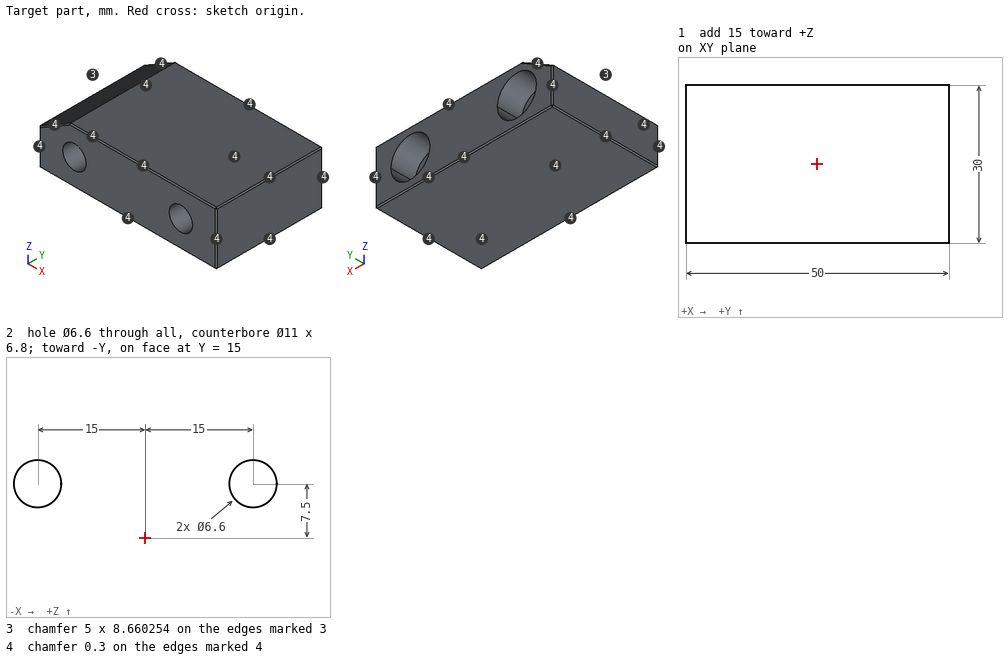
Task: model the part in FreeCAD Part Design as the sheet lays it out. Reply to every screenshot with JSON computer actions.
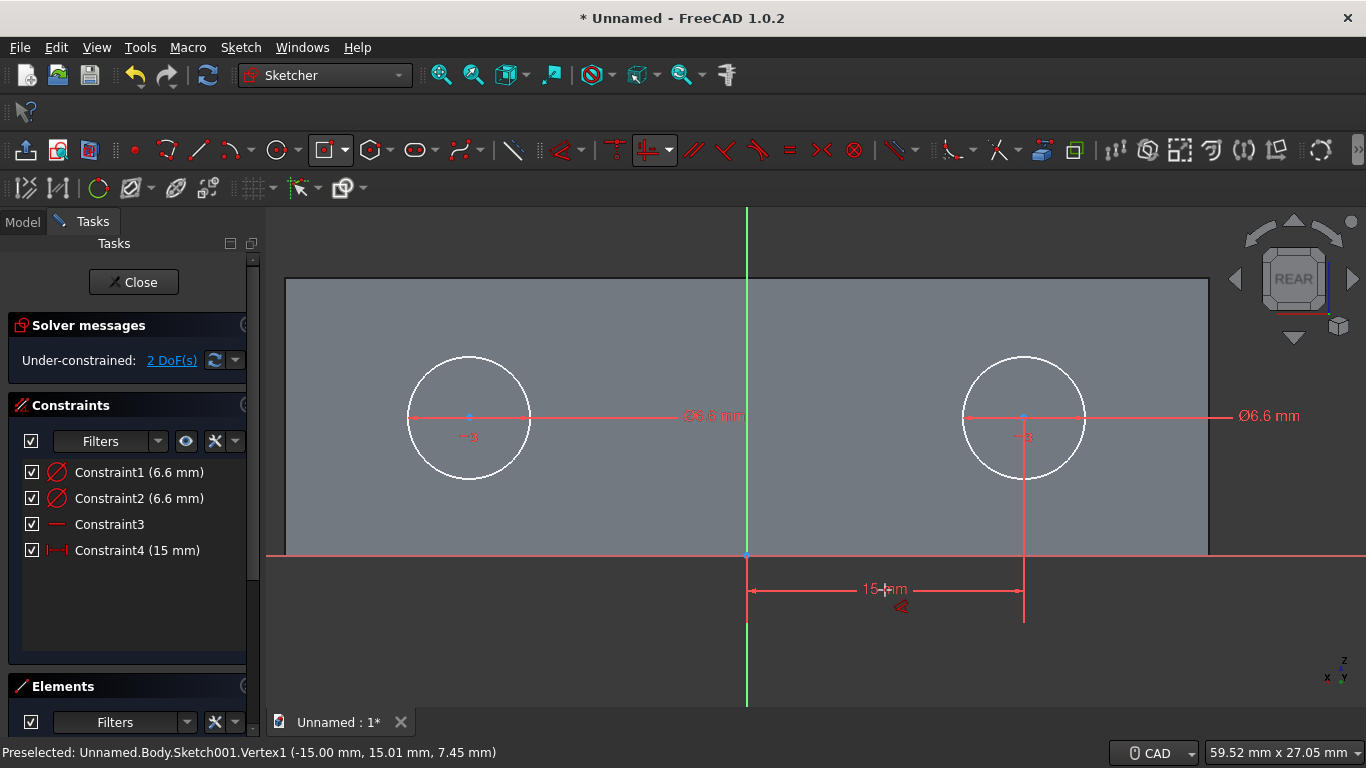
{"action": "left_click", "coordinate": [469, 418]}
{"action": "left_click", "coordinate": [608, 590]}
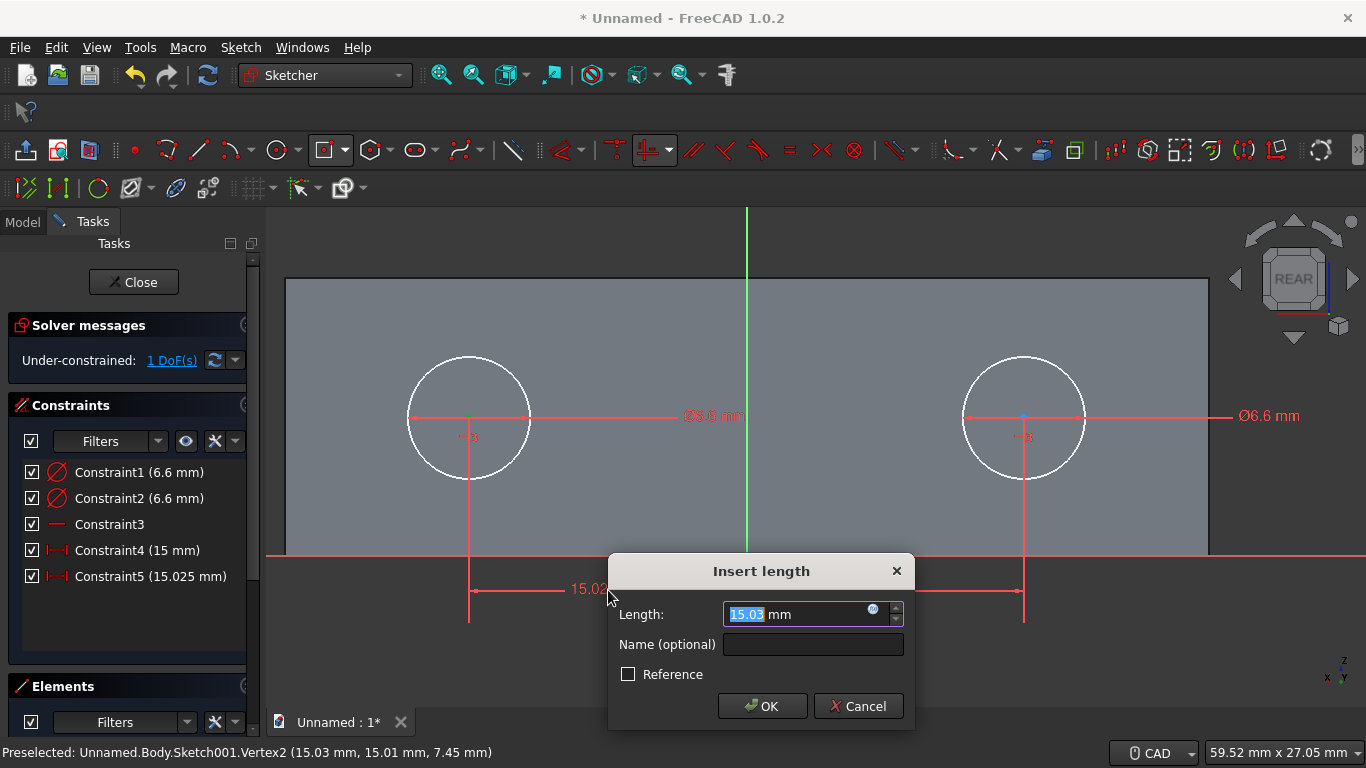
{"action": "type", "text": "15"}
{"action": "key", "text": "Return"}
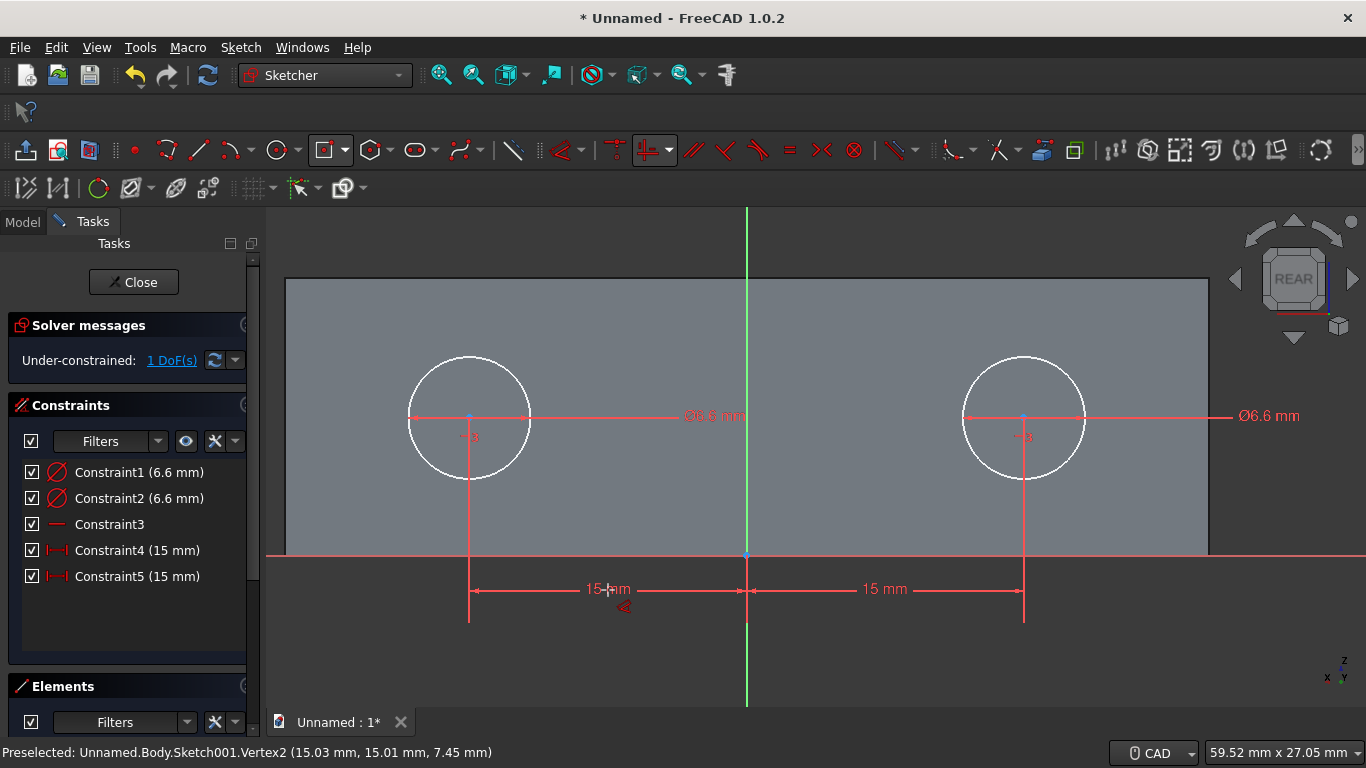
{"action": "left_click", "coordinate": [1024, 418]}
{"action": "left_click", "coordinate": [1058, 487]}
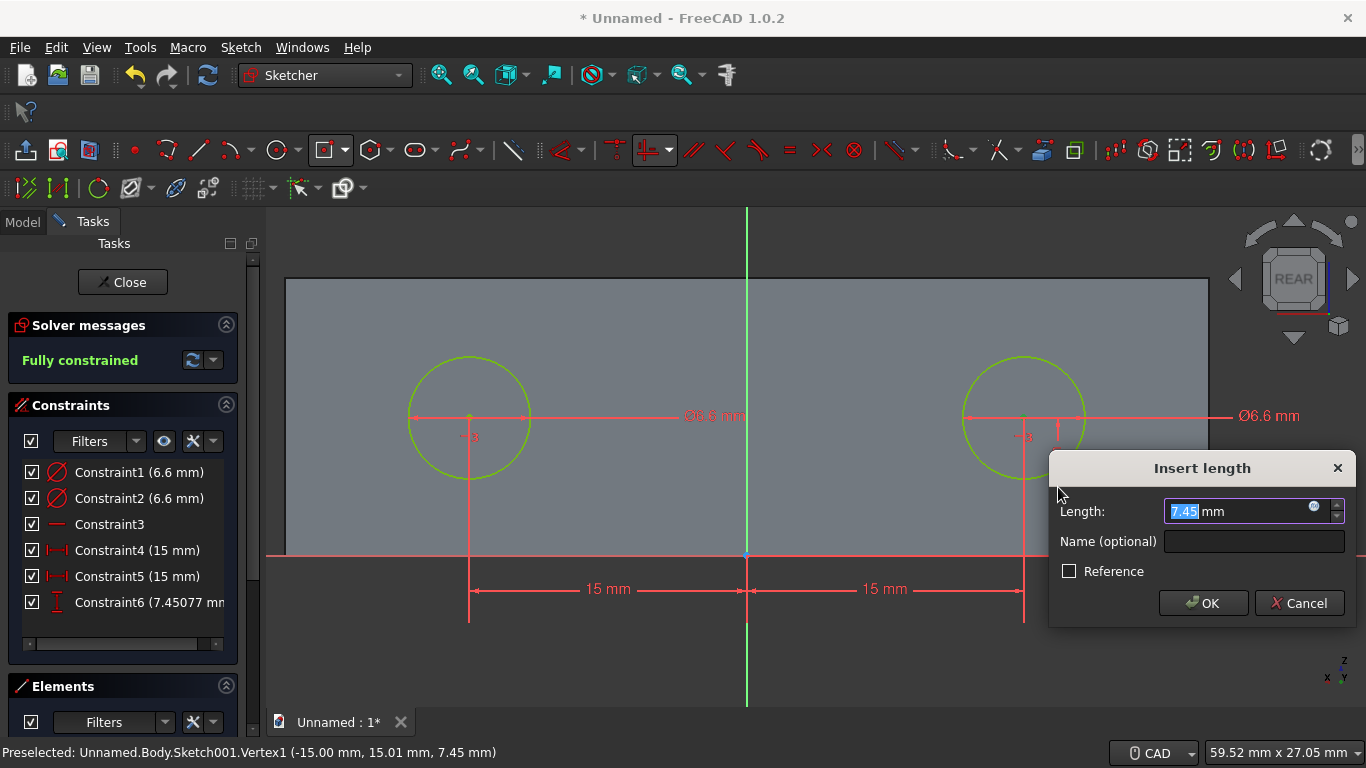
{"action": "type", "text": "7.5"}
{"action": "key", "text": "Return"}
{"action": "key", "text": "Escape"}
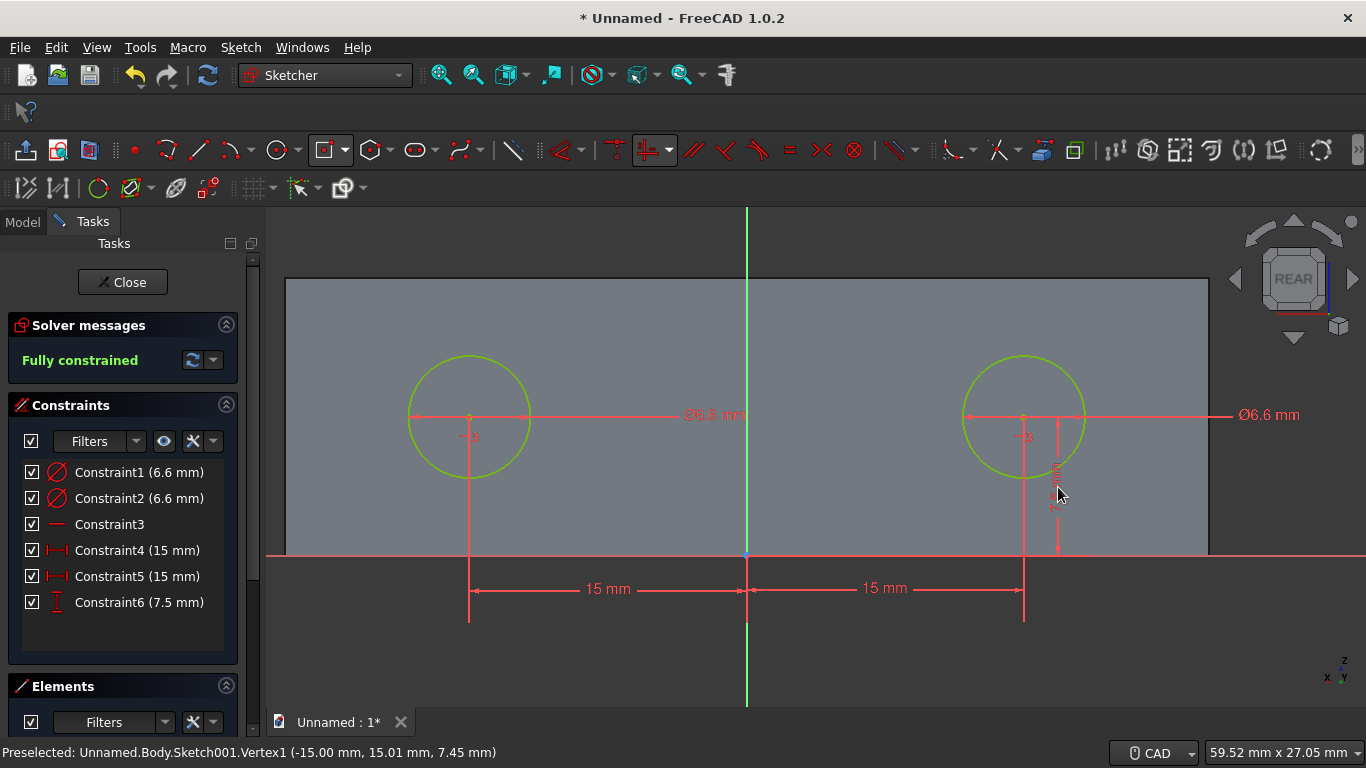
{"action": "left_click", "coordinate": [123, 282]}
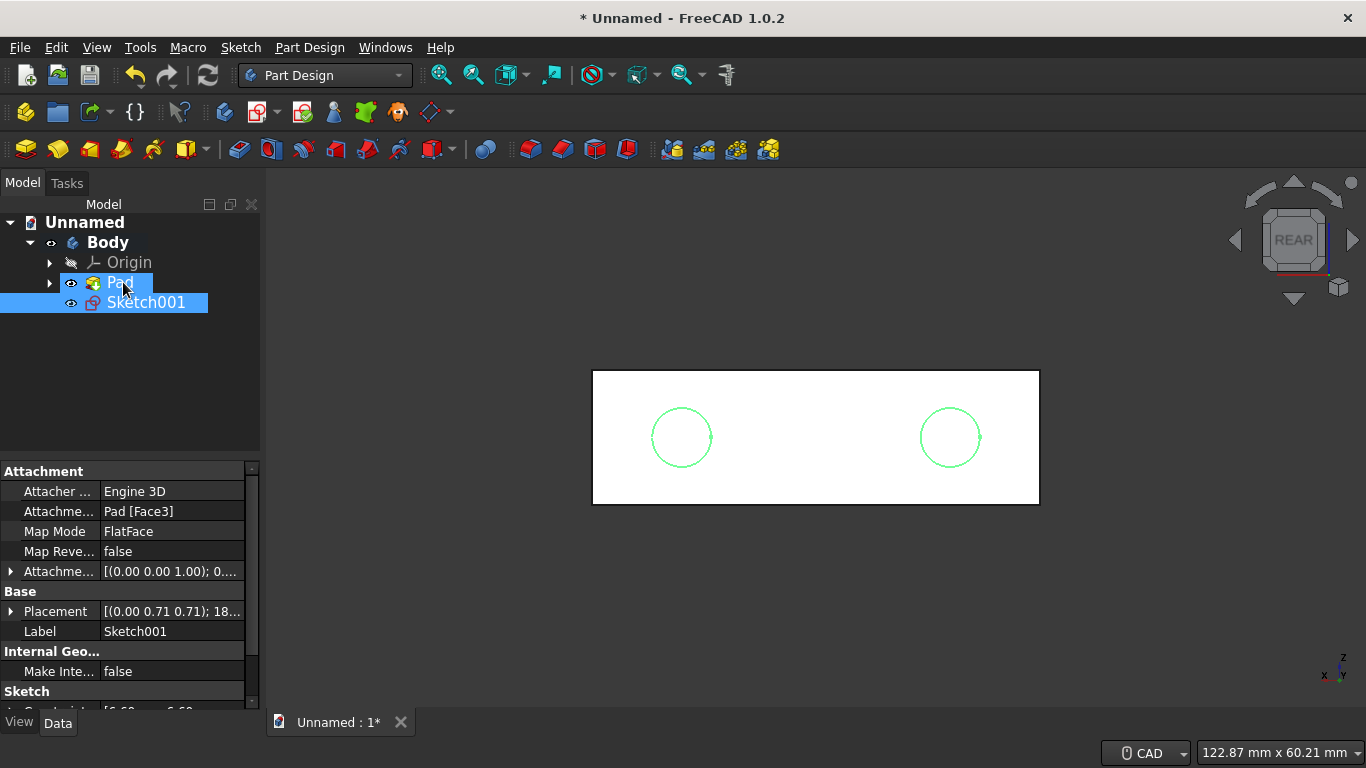
{"action": "left_click", "coordinate": [272, 150]}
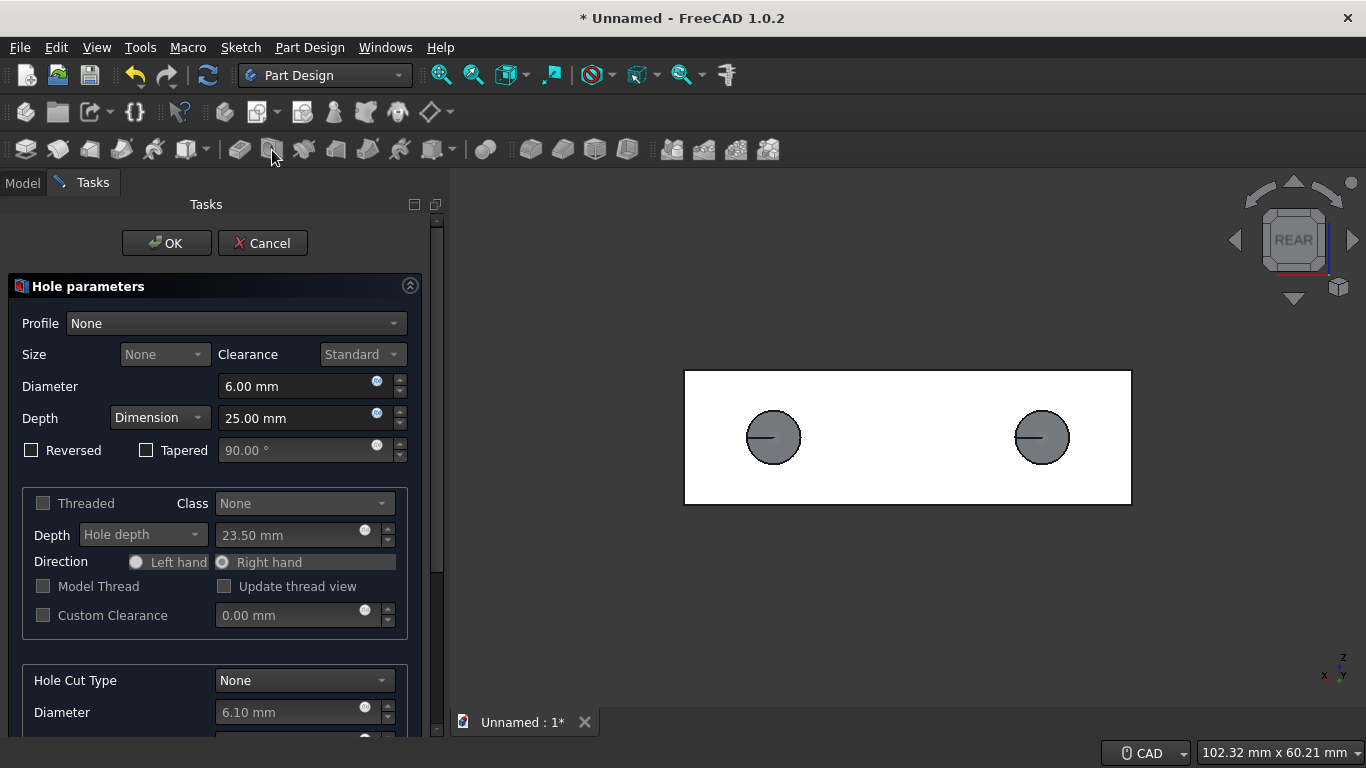
{"action": "triple_click", "coordinate": [305, 386]}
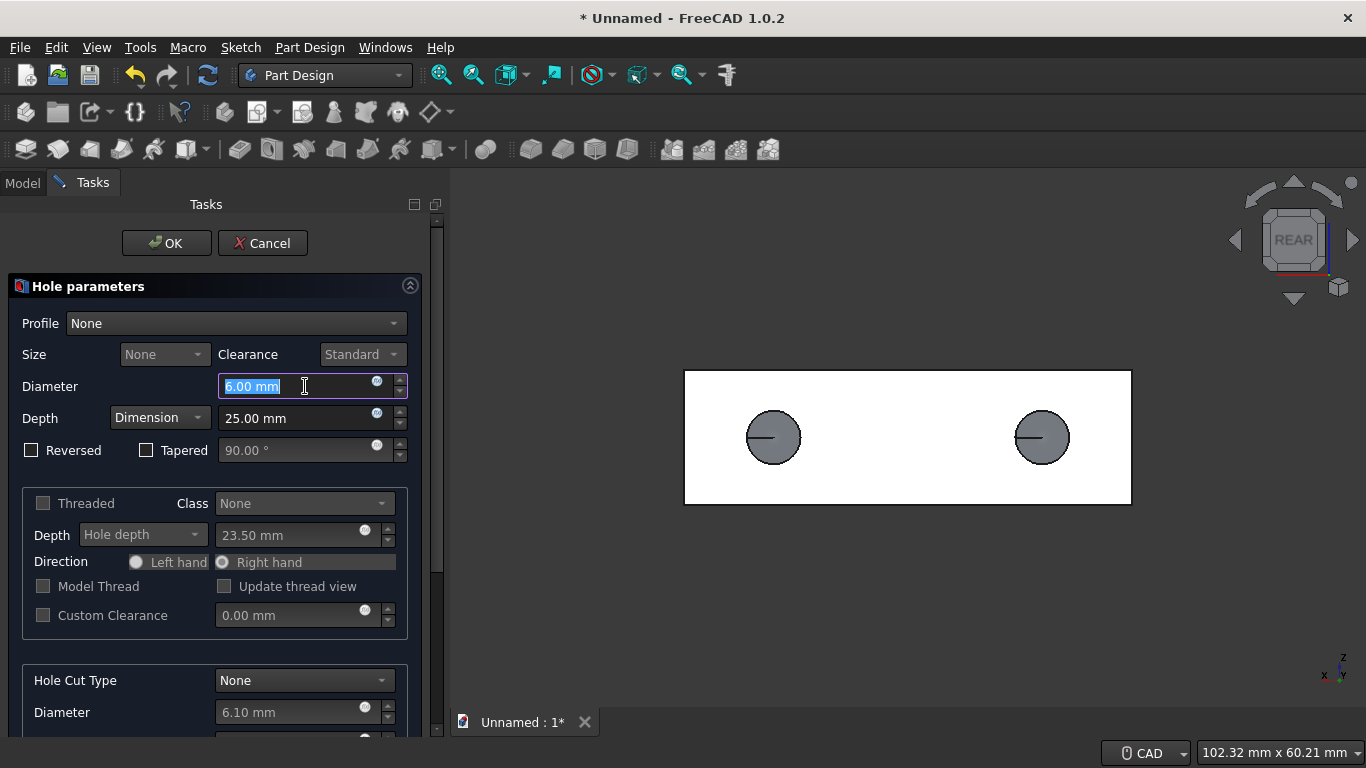
{"action": "type", "text": "6.6"}
{"action": "key", "text": "Tab"}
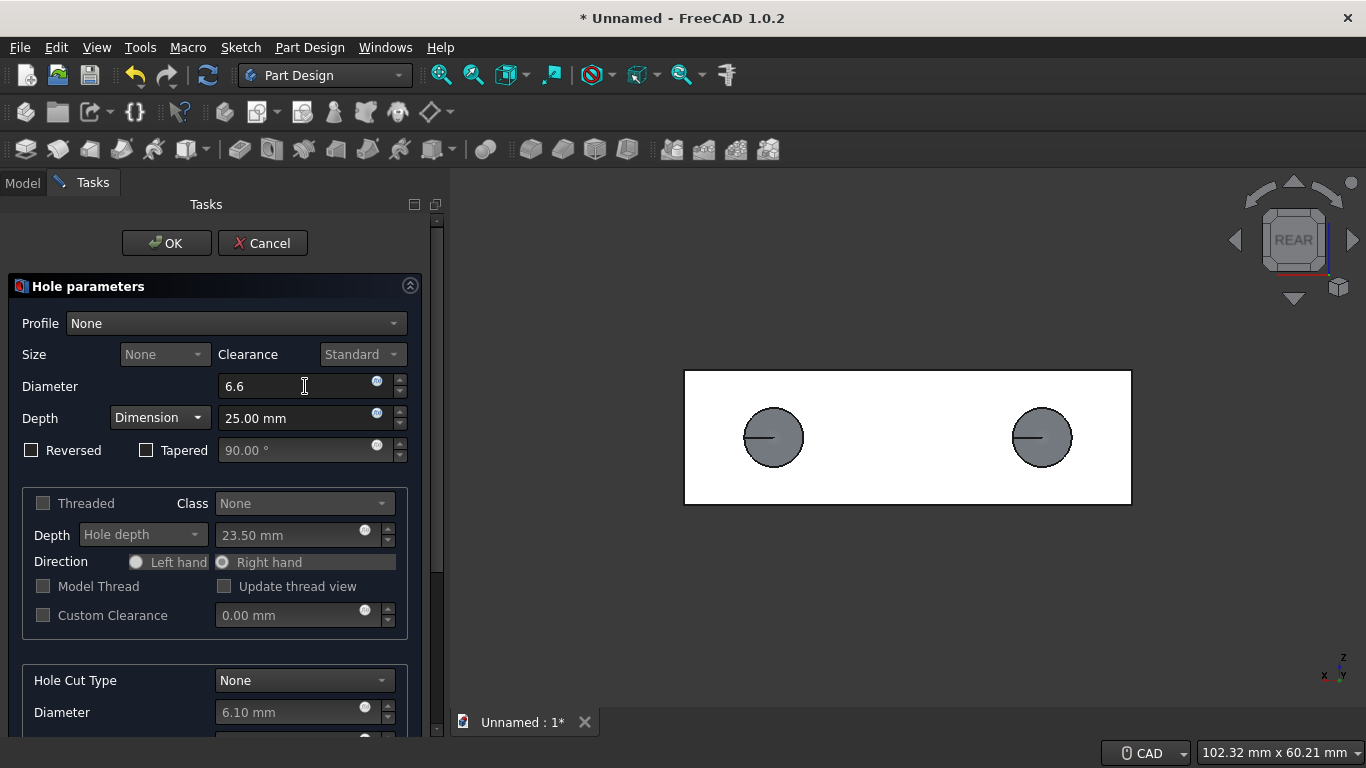
{"action": "left_click", "coordinate": [161, 418]}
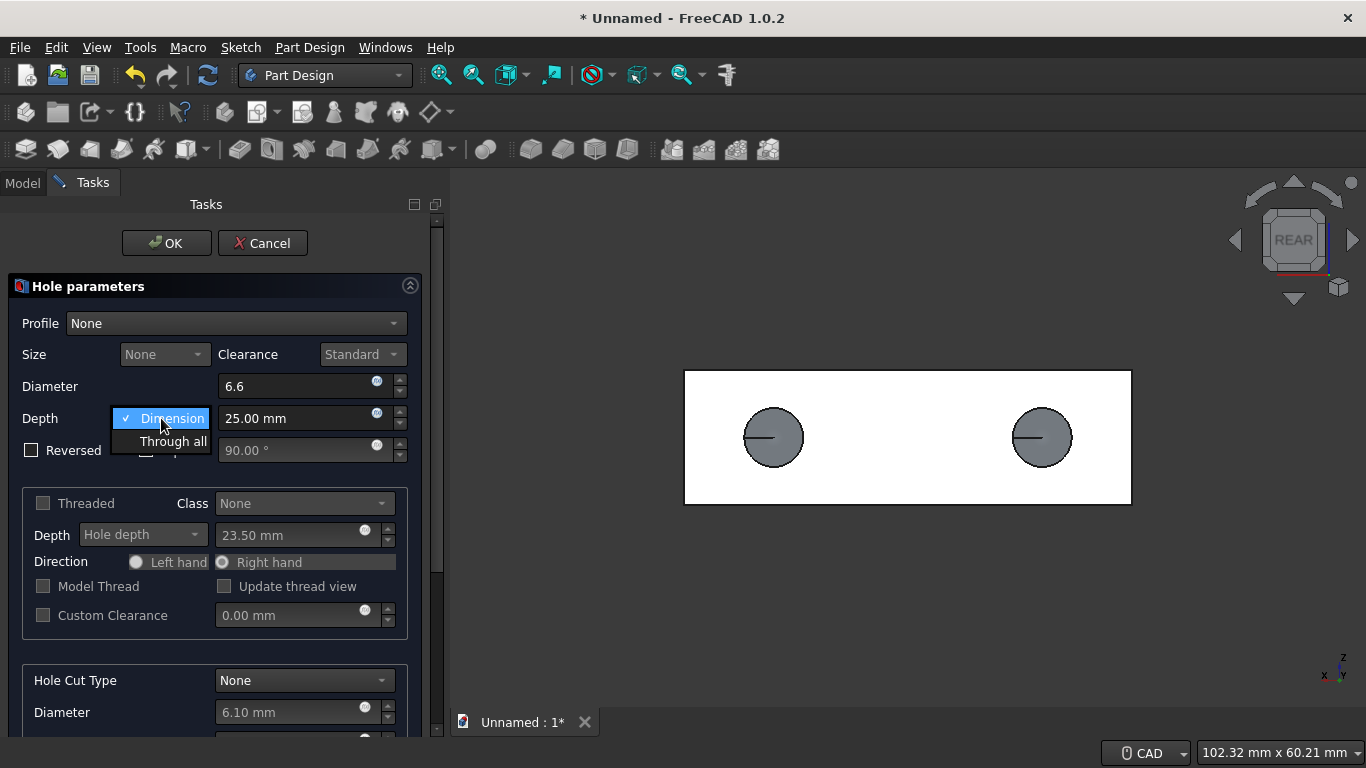
{"action": "left_click", "coordinate": [160, 442]}